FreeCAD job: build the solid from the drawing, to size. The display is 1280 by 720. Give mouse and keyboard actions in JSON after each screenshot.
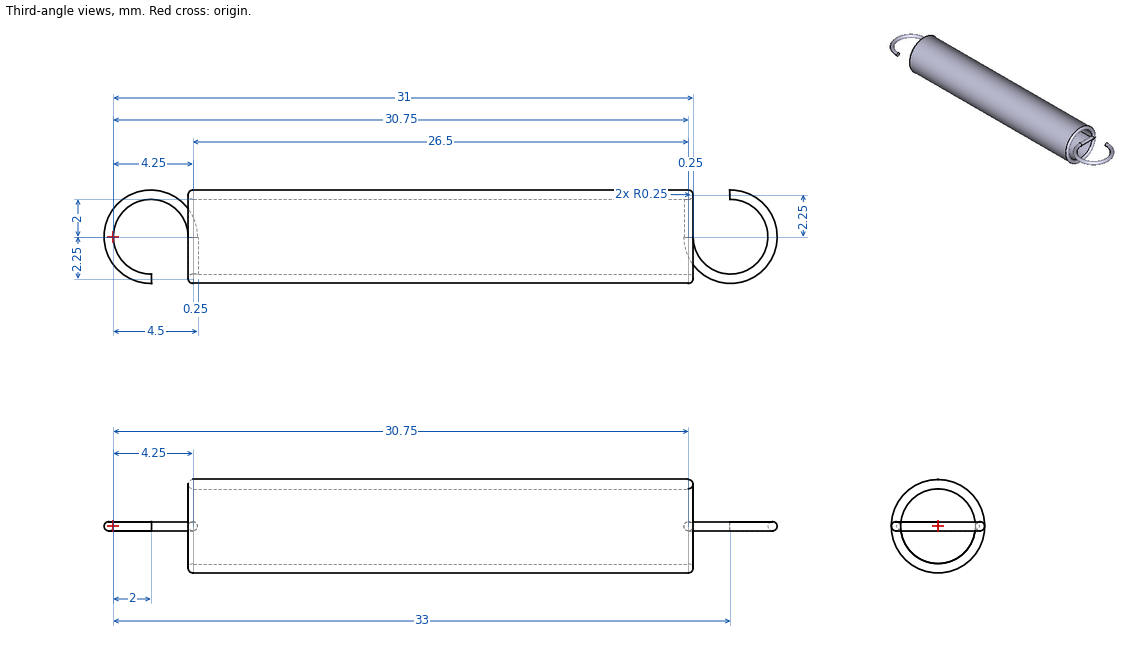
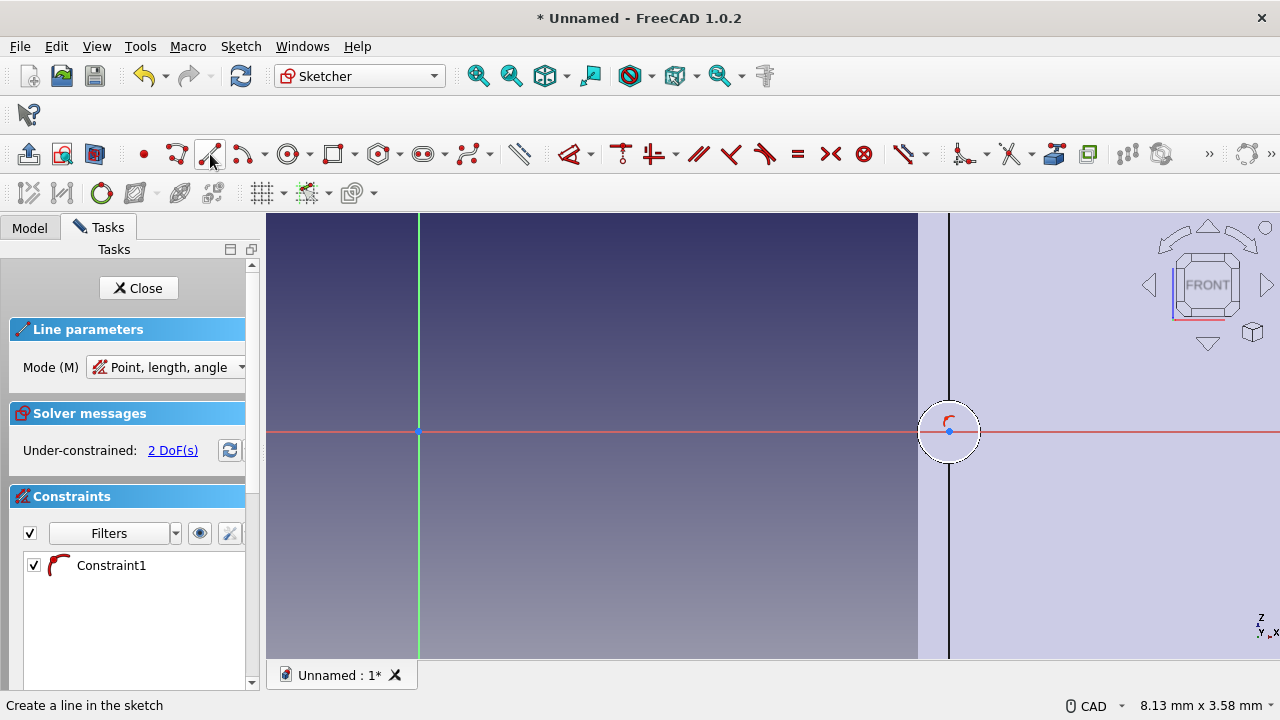
{"action": "left_click", "coordinate": [668, 469]}
{"action": "left_click", "coordinate": [668, 395]}
{"action": "key", "text": "Escape"}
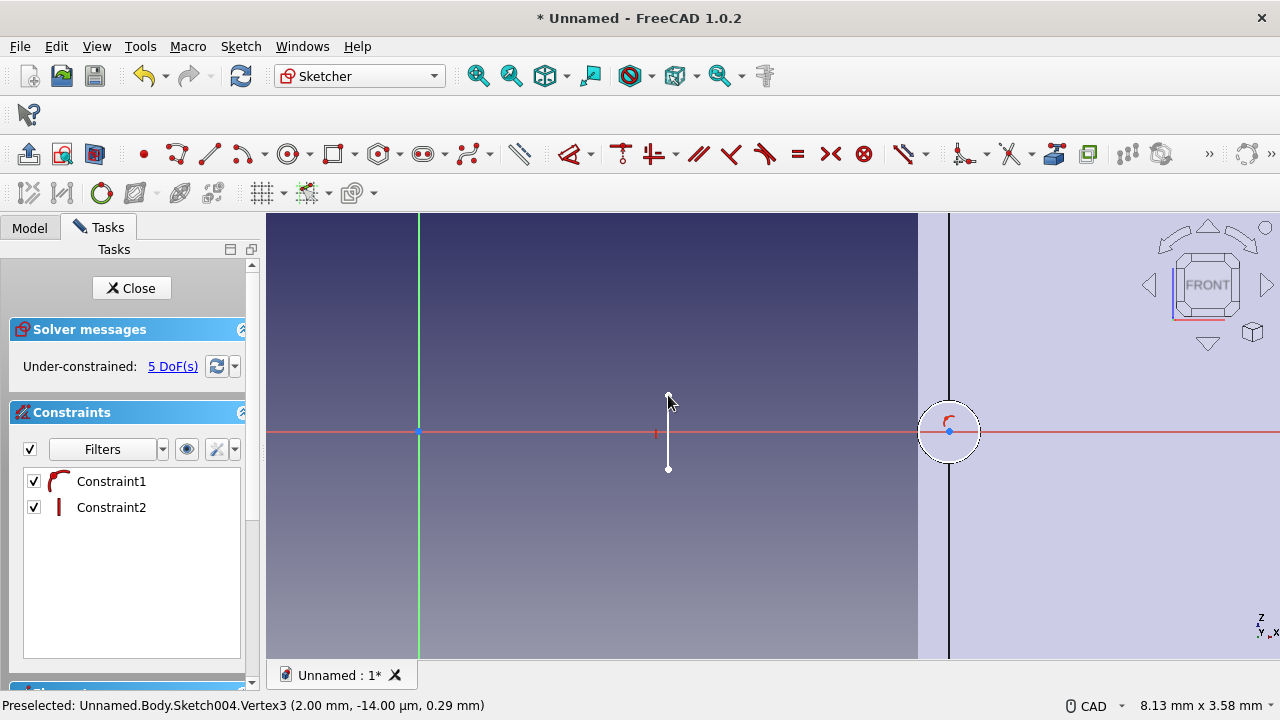
{"action": "left_click", "coordinate": [668, 448]}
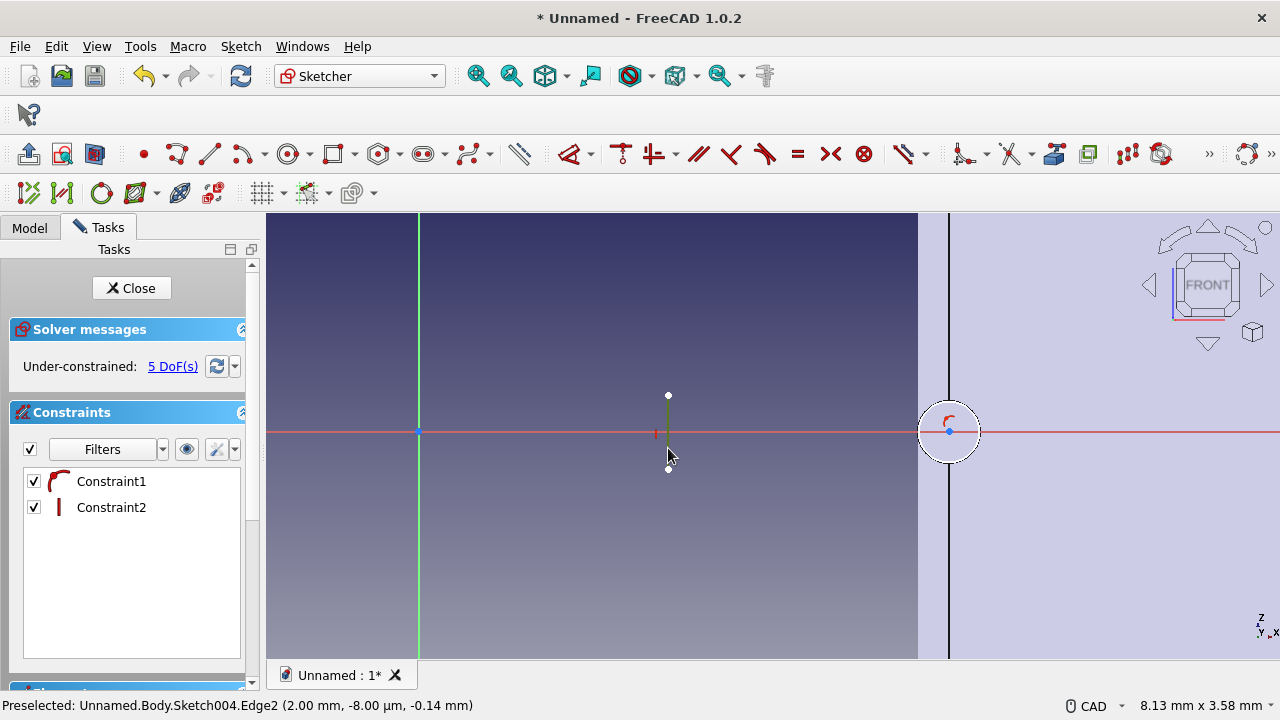
{"action": "left_click", "coordinate": [520, 154]}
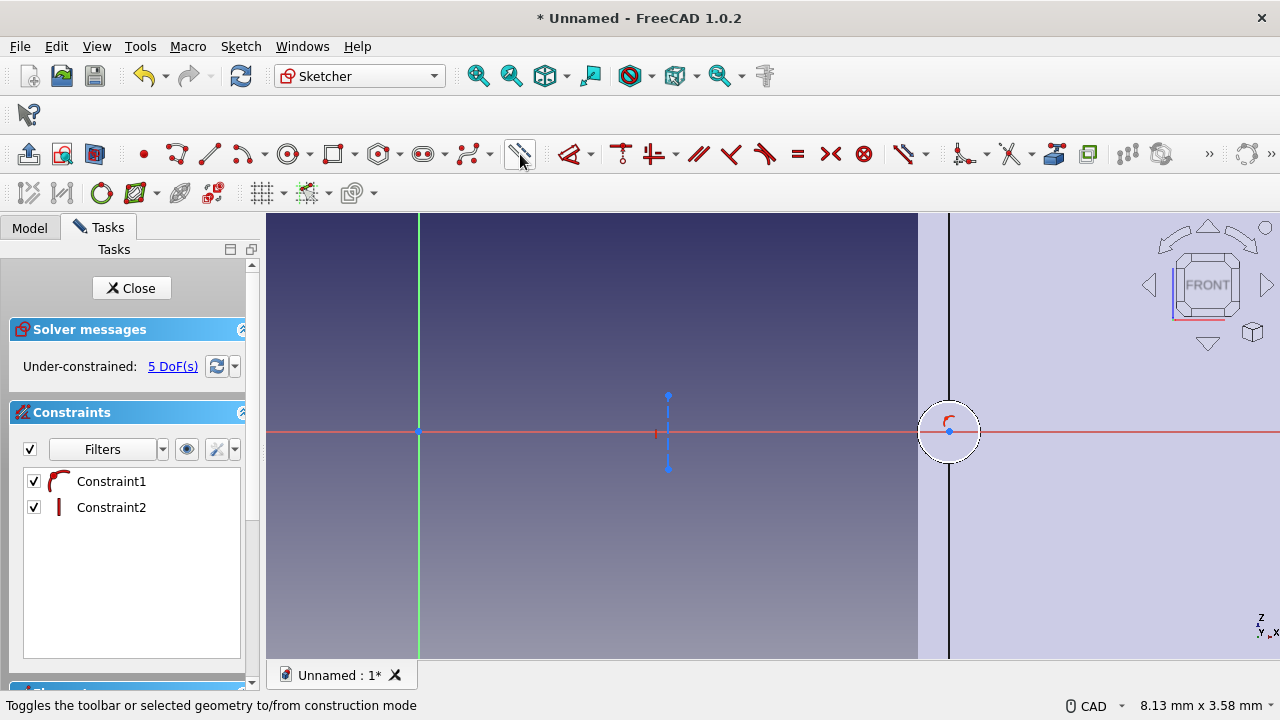
{"action": "key", "text": "d"}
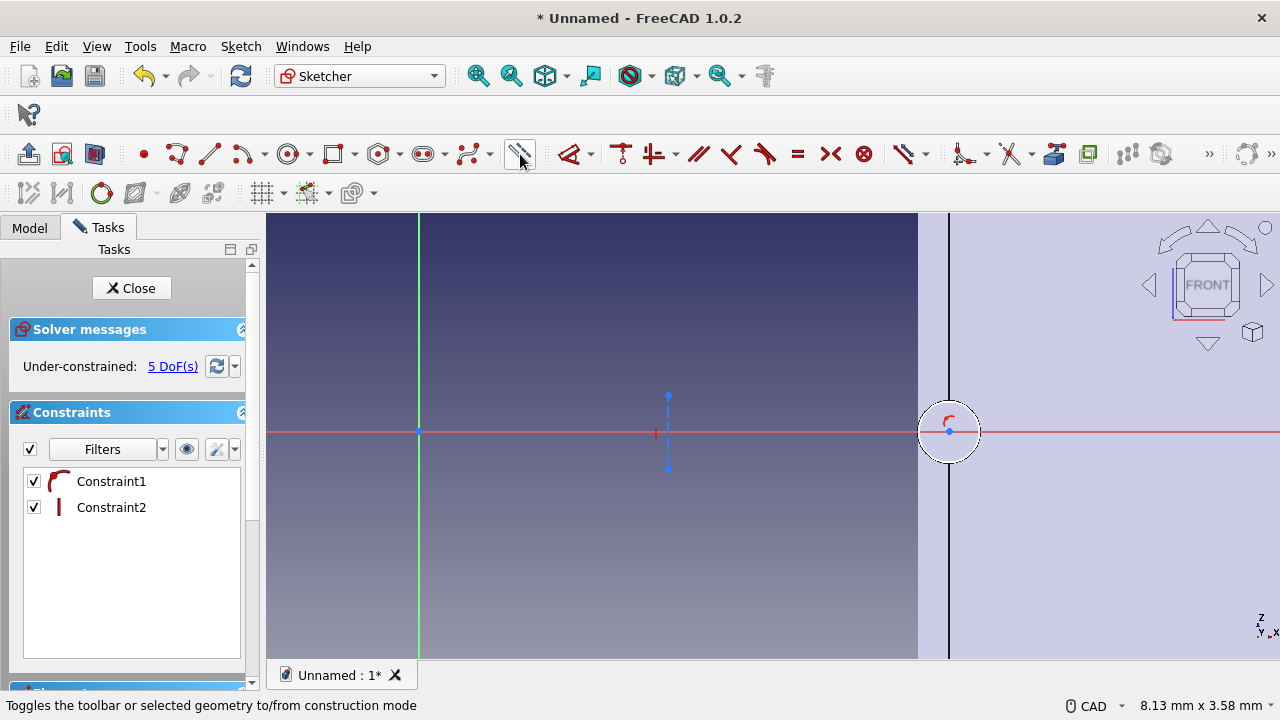
{"action": "left_click", "coordinate": [970, 410]}
{"action": "left_click", "coordinate": [992, 387]}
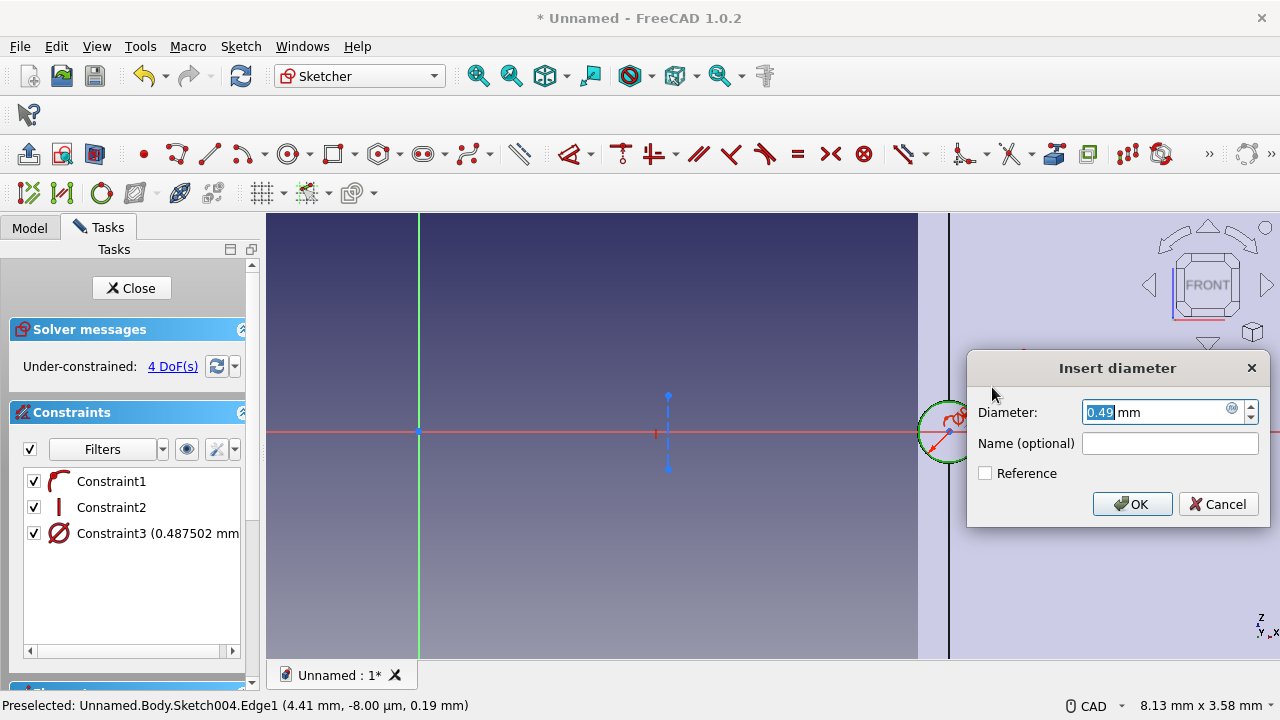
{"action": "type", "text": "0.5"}
{"action": "key", "text": "Return"}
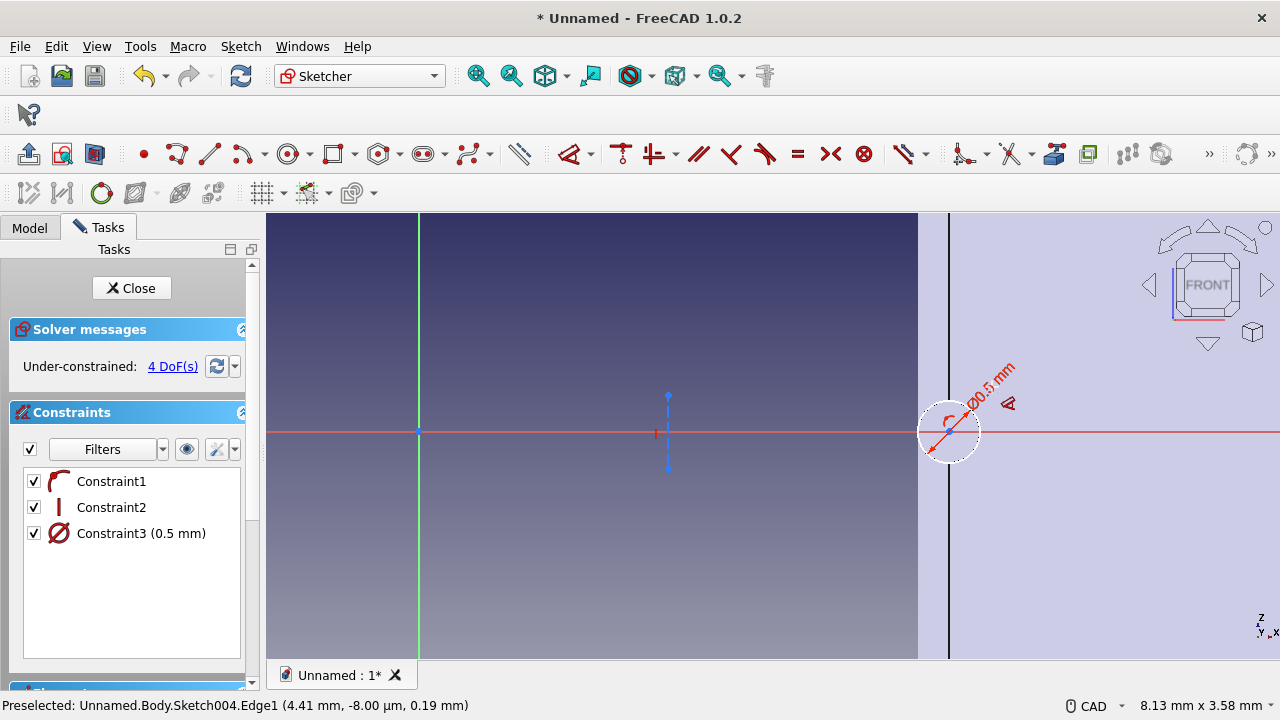
{"action": "left_click", "coordinate": [668, 470]}
{"action": "left_click", "coordinate": [543, 504]}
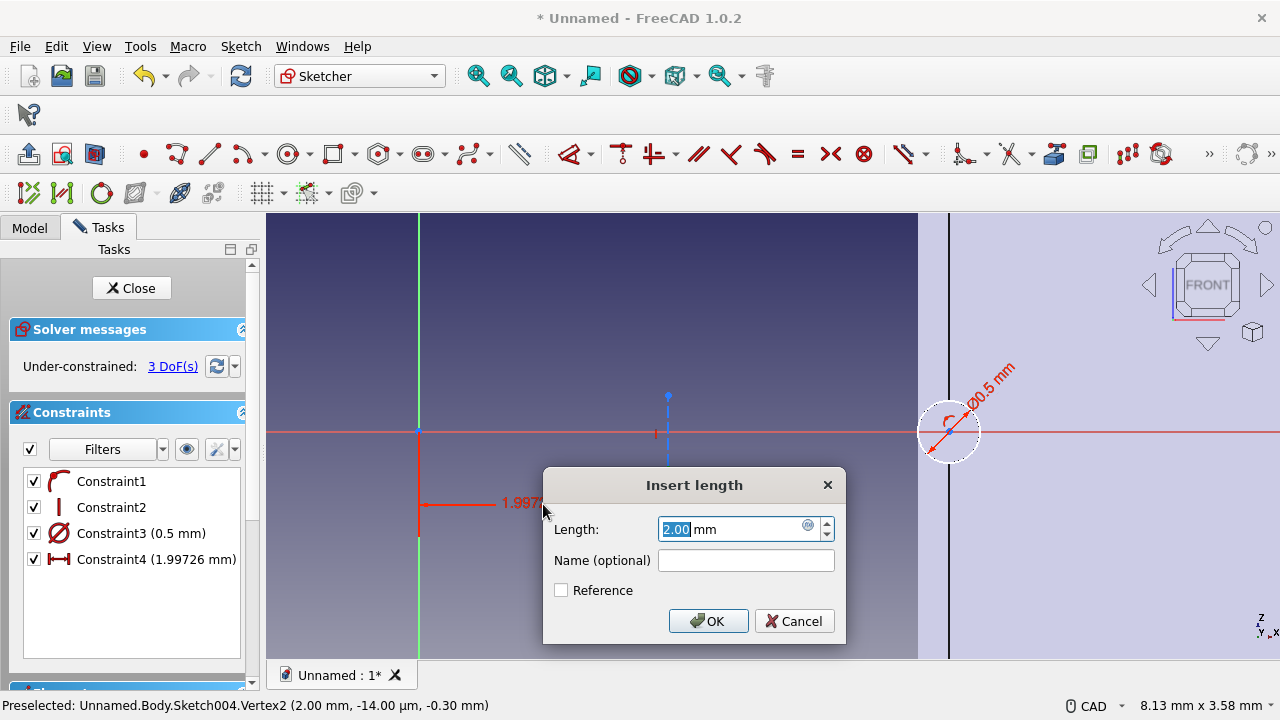
{"action": "type", "text": "2"}
{"action": "key", "text": "Return"}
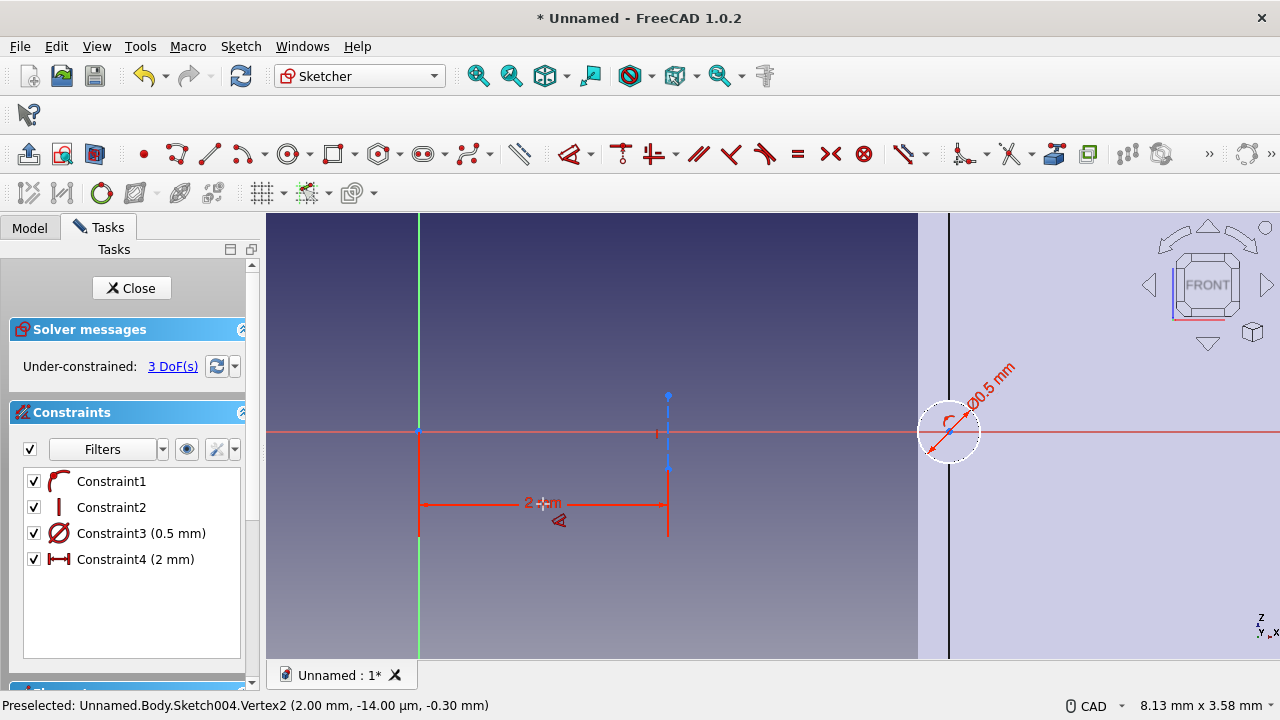
{"action": "left_click", "coordinate": [949, 432]}
{"action": "left_click", "coordinate": [684, 466]}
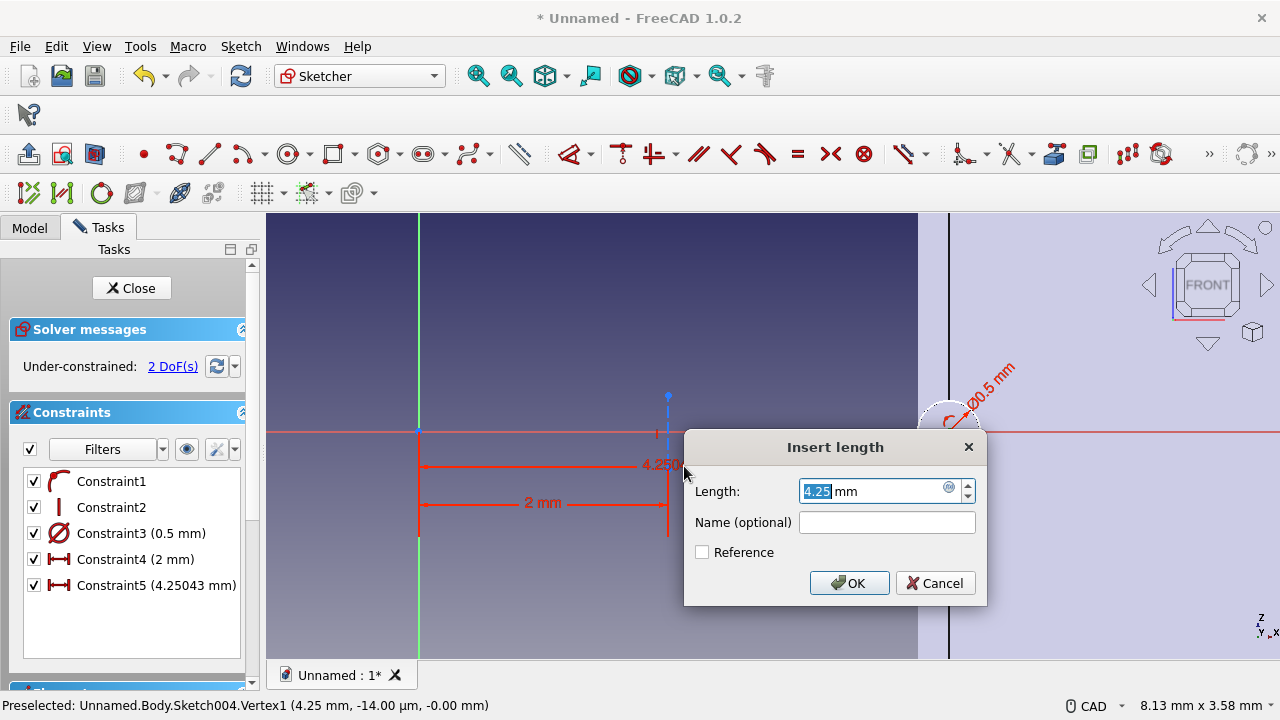
{"action": "type", "text": "4.25"}
{"action": "key", "text": "Return"}
{"action": "key", "text": "Escape"}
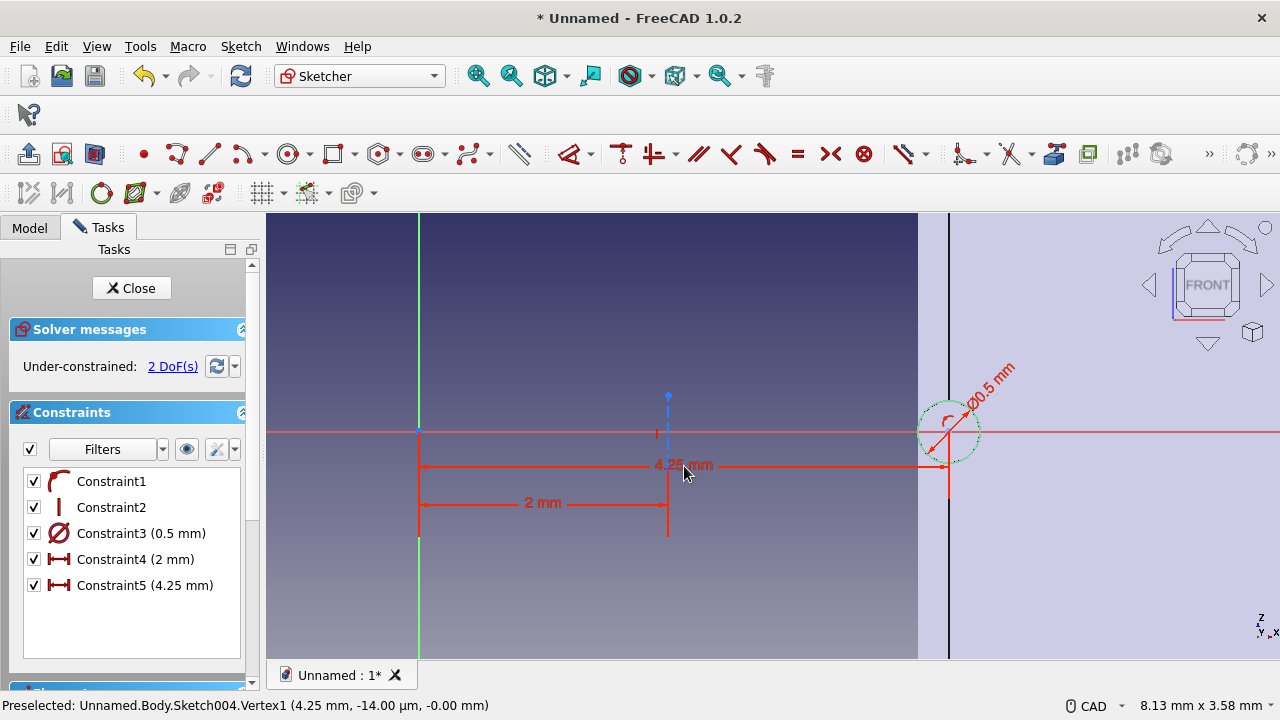
{"action": "left_click", "coordinate": [132, 288]}